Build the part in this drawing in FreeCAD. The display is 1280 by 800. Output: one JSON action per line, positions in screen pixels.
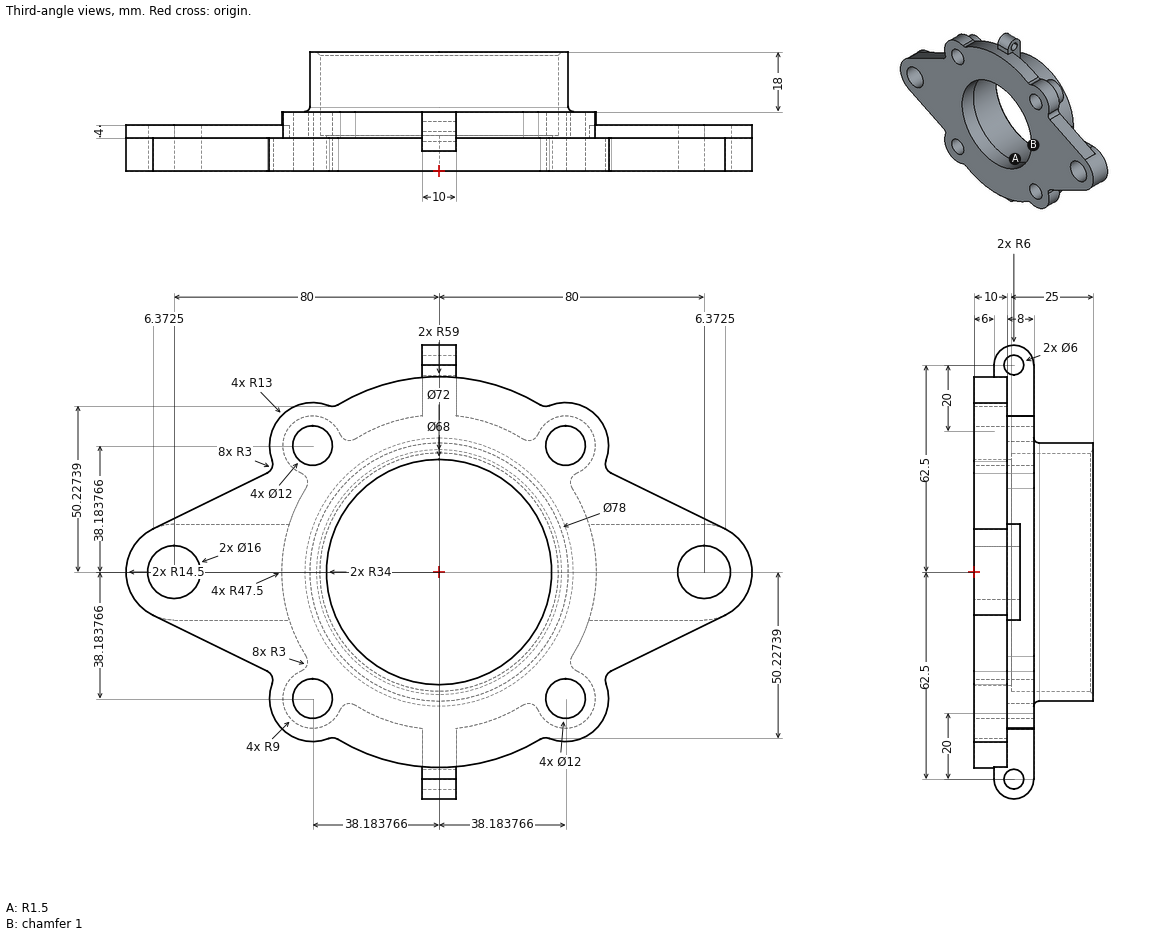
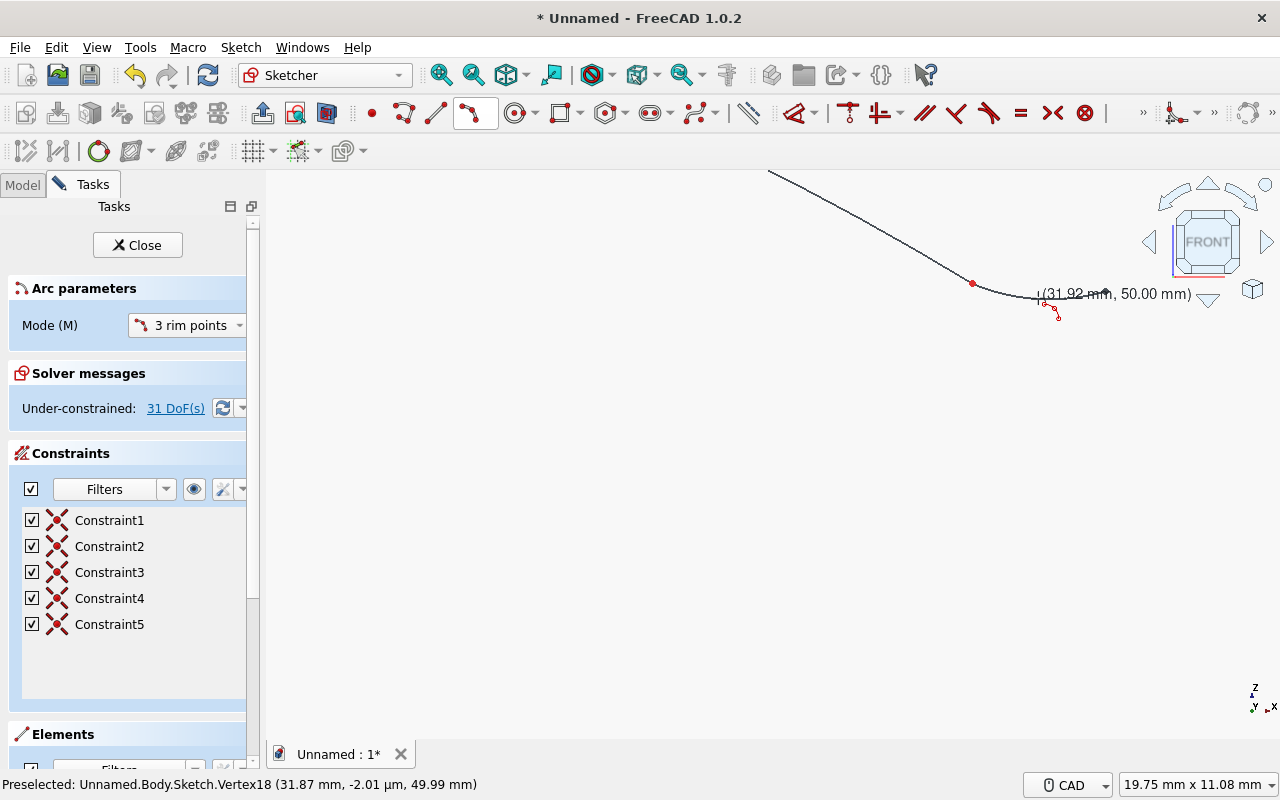
{"action": "scroll", "coordinate": [789, 298], "scroll_direction": "down", "scroll_amount": 14}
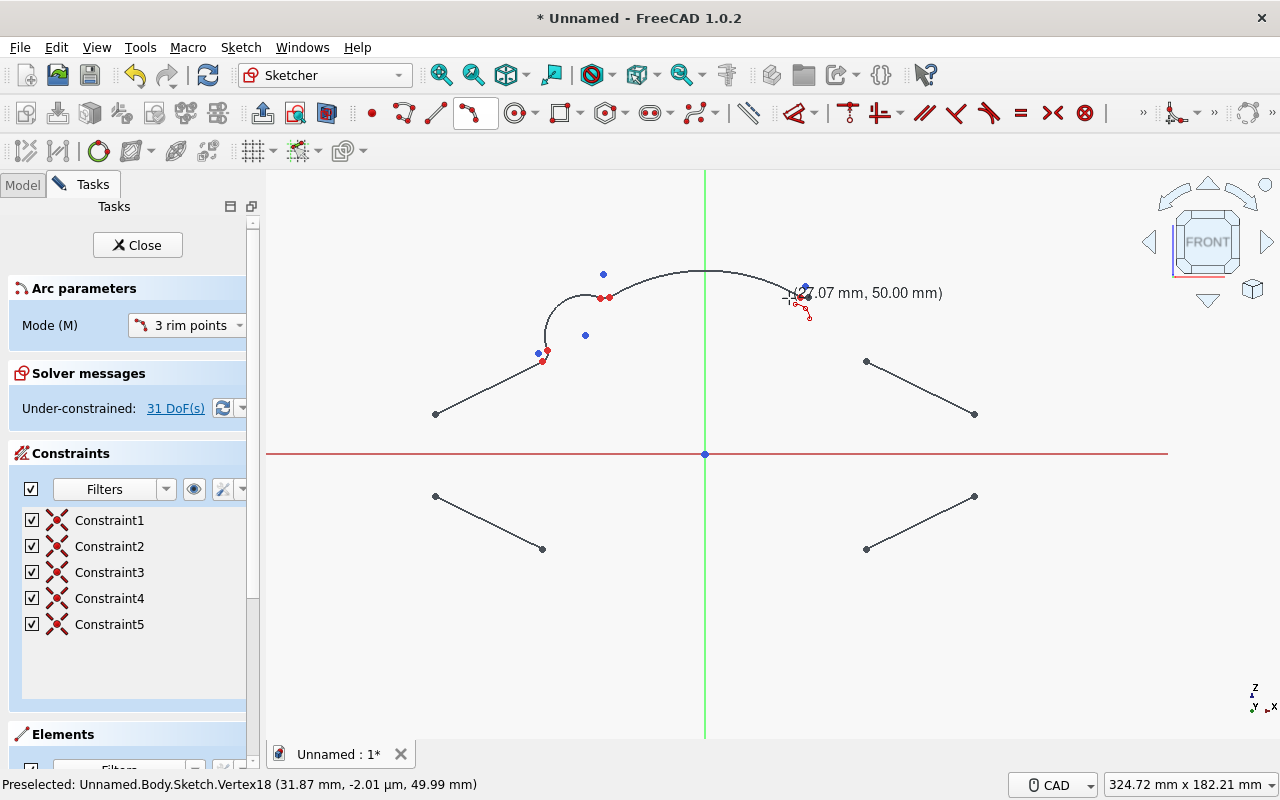
{"action": "scroll", "coordinate": [809, 298], "scroll_direction": "up", "scroll_amount": 4}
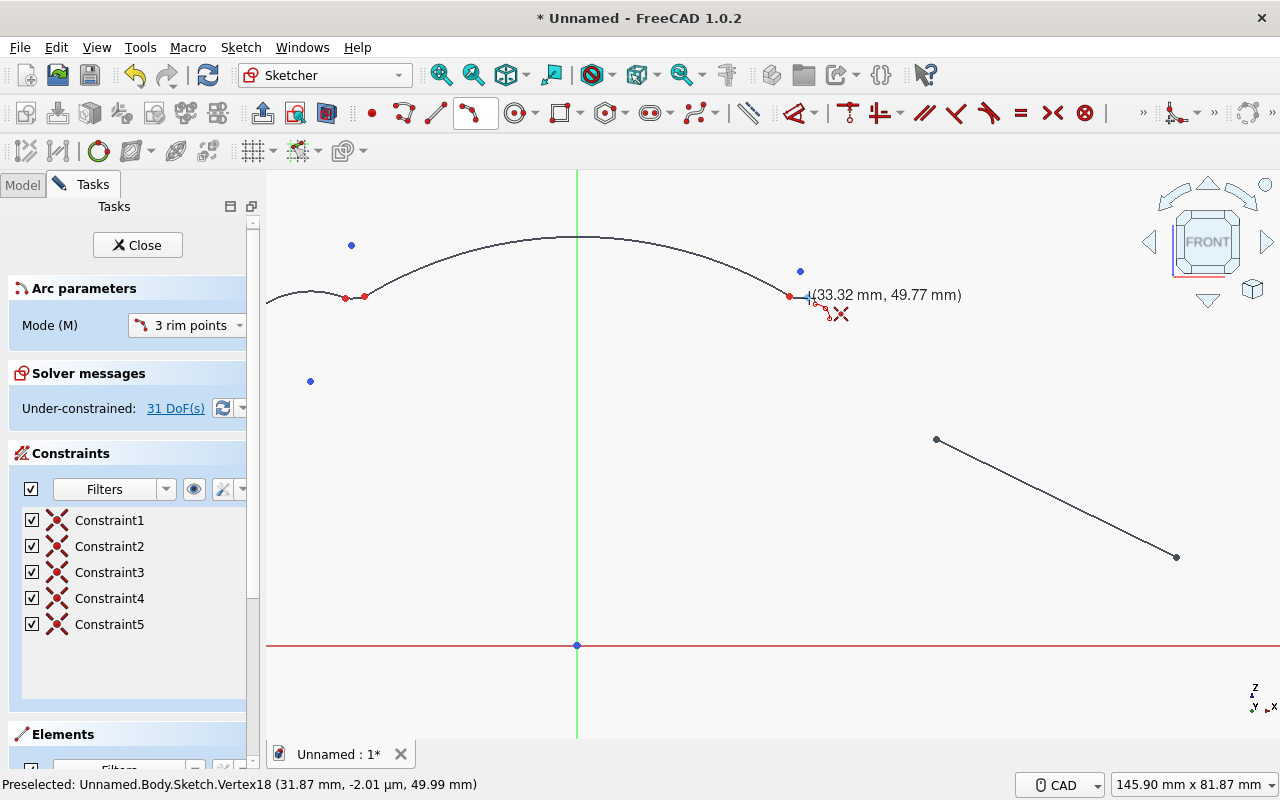
{"action": "left_click", "coordinate": [808, 297]}
{"action": "left_click", "coordinate": [927, 412]}
{"action": "left_click", "coordinate": [905, 316]}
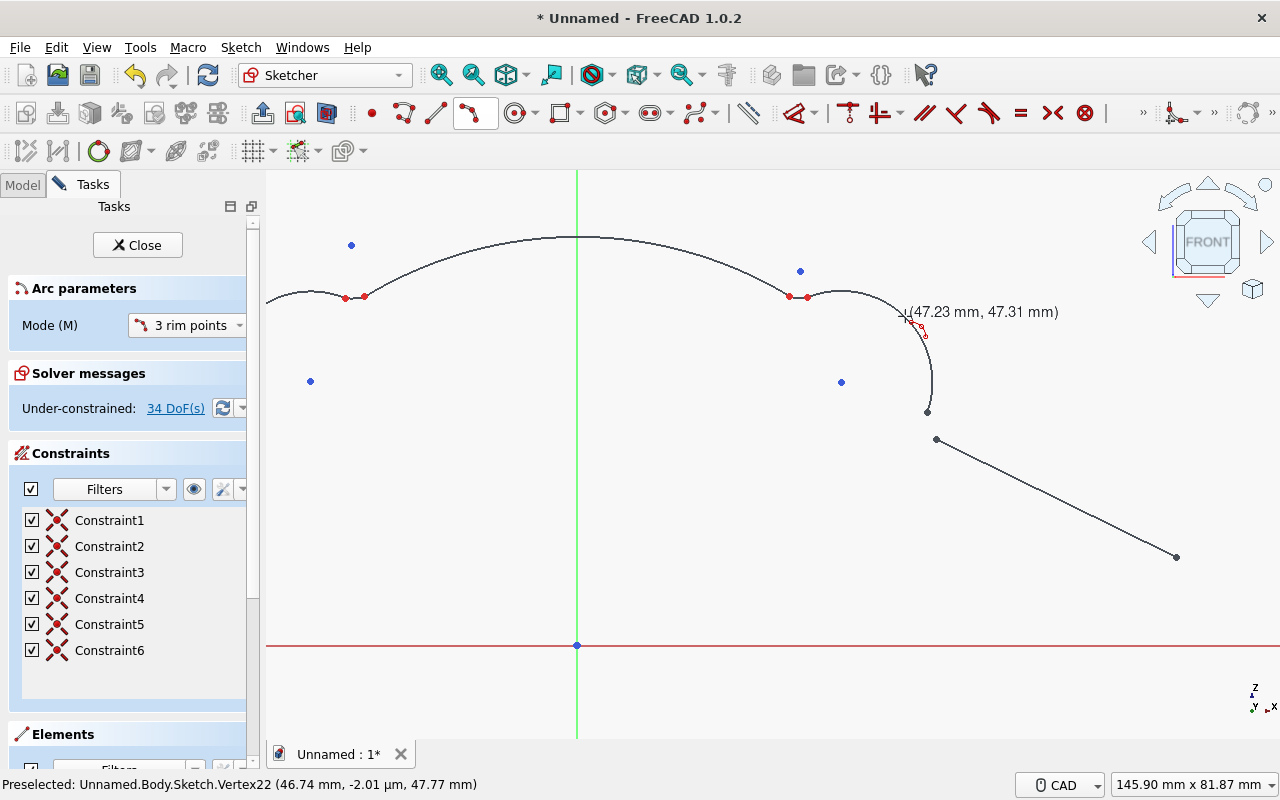
{"action": "left_click", "coordinate": [927, 413]}
{"action": "left_click", "coordinate": [937, 440]}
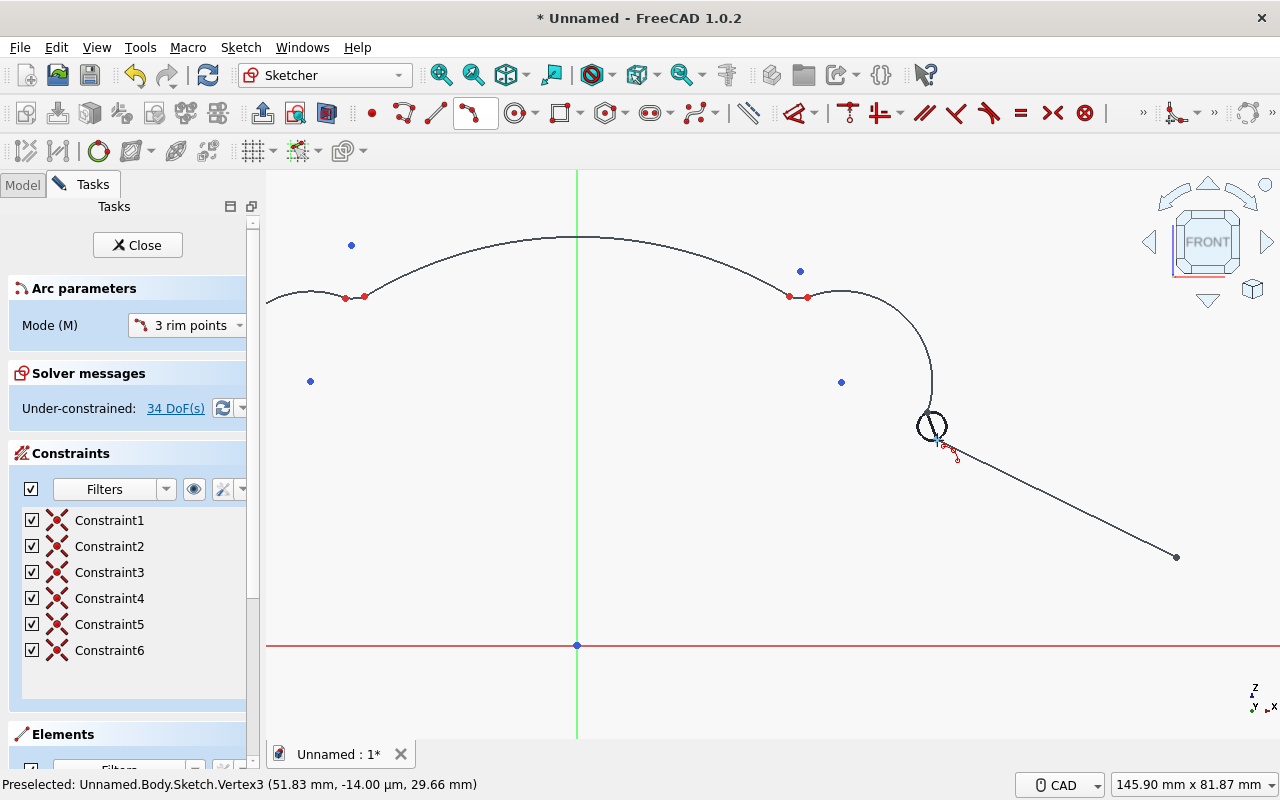
{"action": "scroll", "coordinate": [927, 427], "scroll_direction": "up", "scroll_amount": 6}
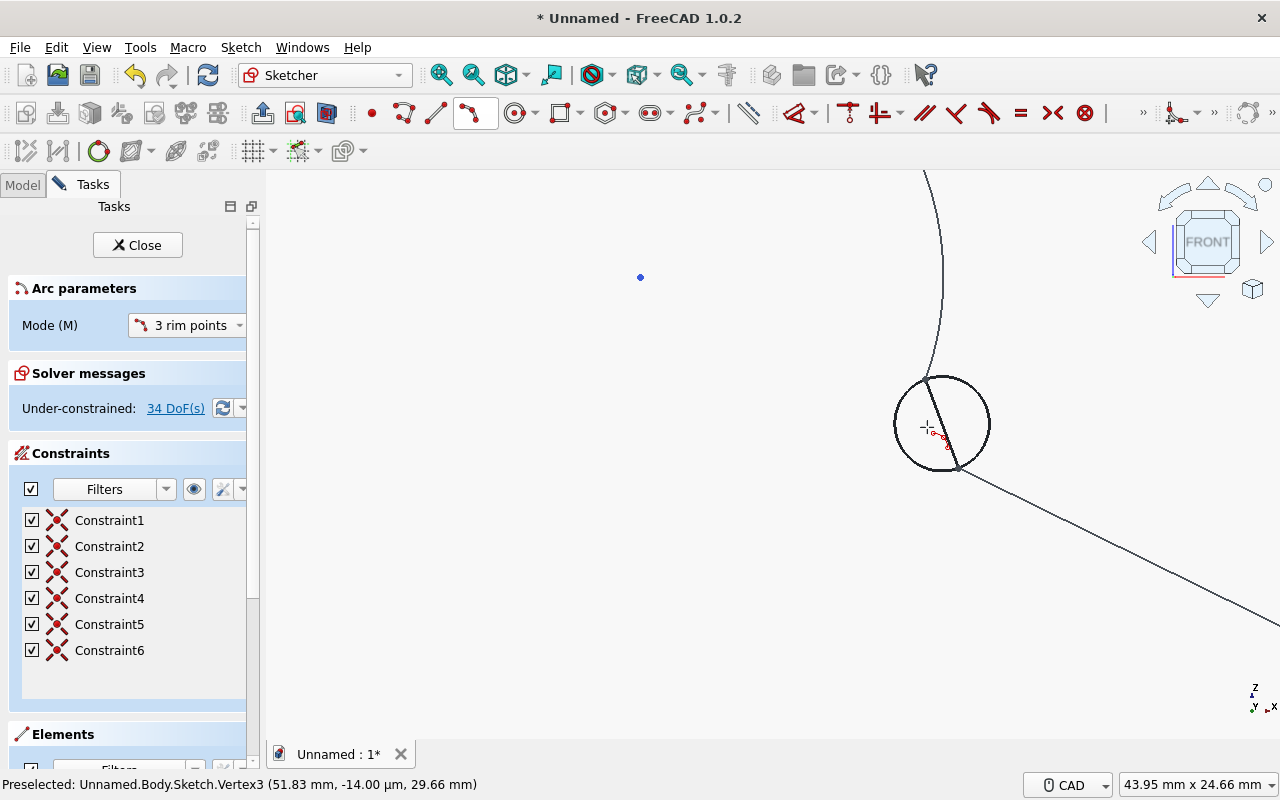
{"action": "left_click", "coordinate": [925, 426]}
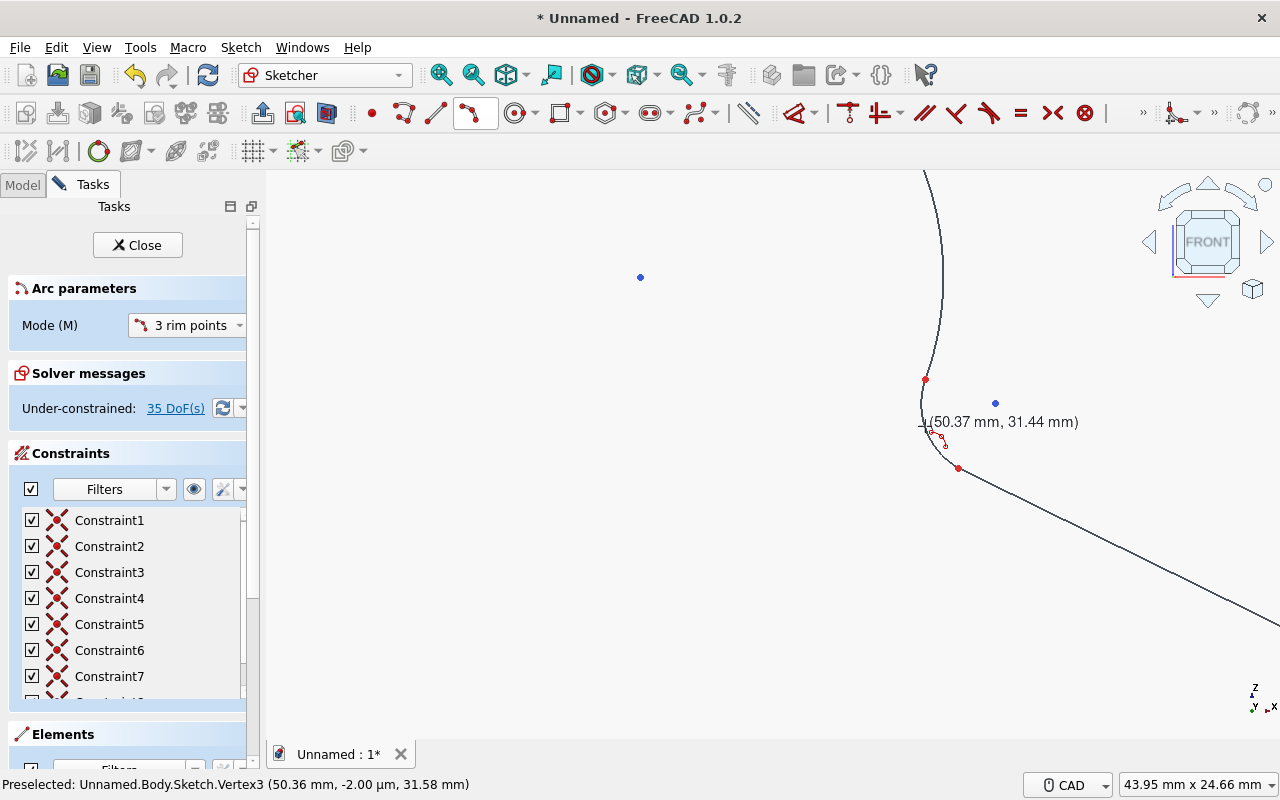
{"action": "scroll", "coordinate": [852, 345], "scroll_direction": "down", "scroll_amount": 10}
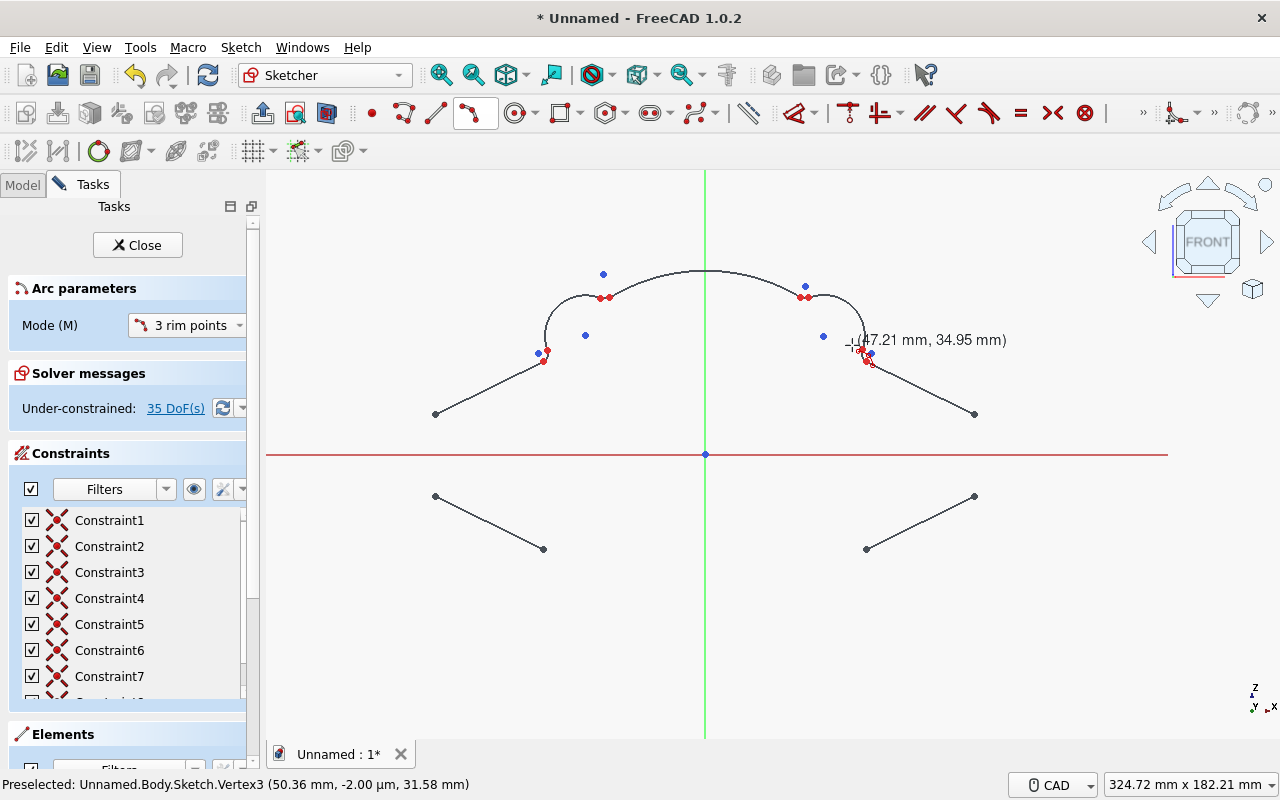
{"action": "left_click", "coordinate": [975, 415]}
{"action": "left_click", "coordinate": [975, 496]}
{"action": "left_click", "coordinate": [996, 474]}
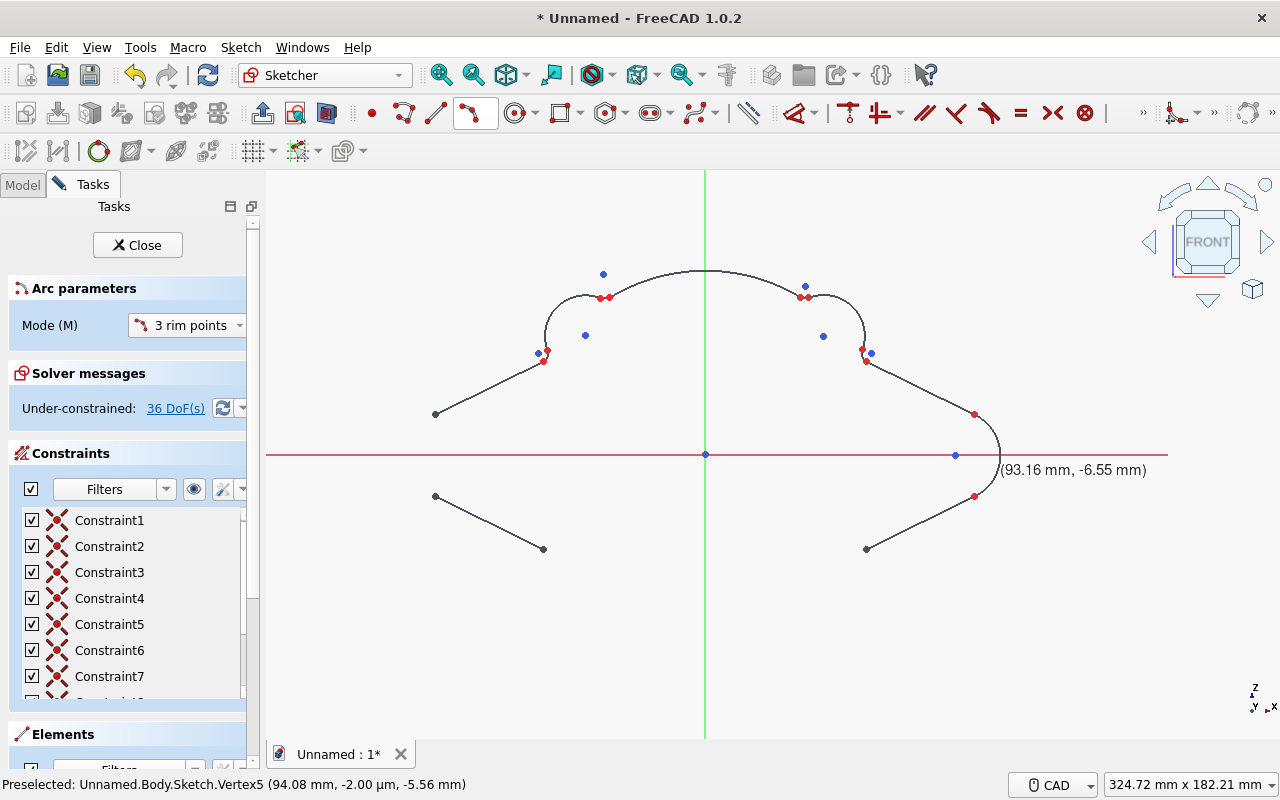
{"action": "left_click", "coordinate": [867, 549]}